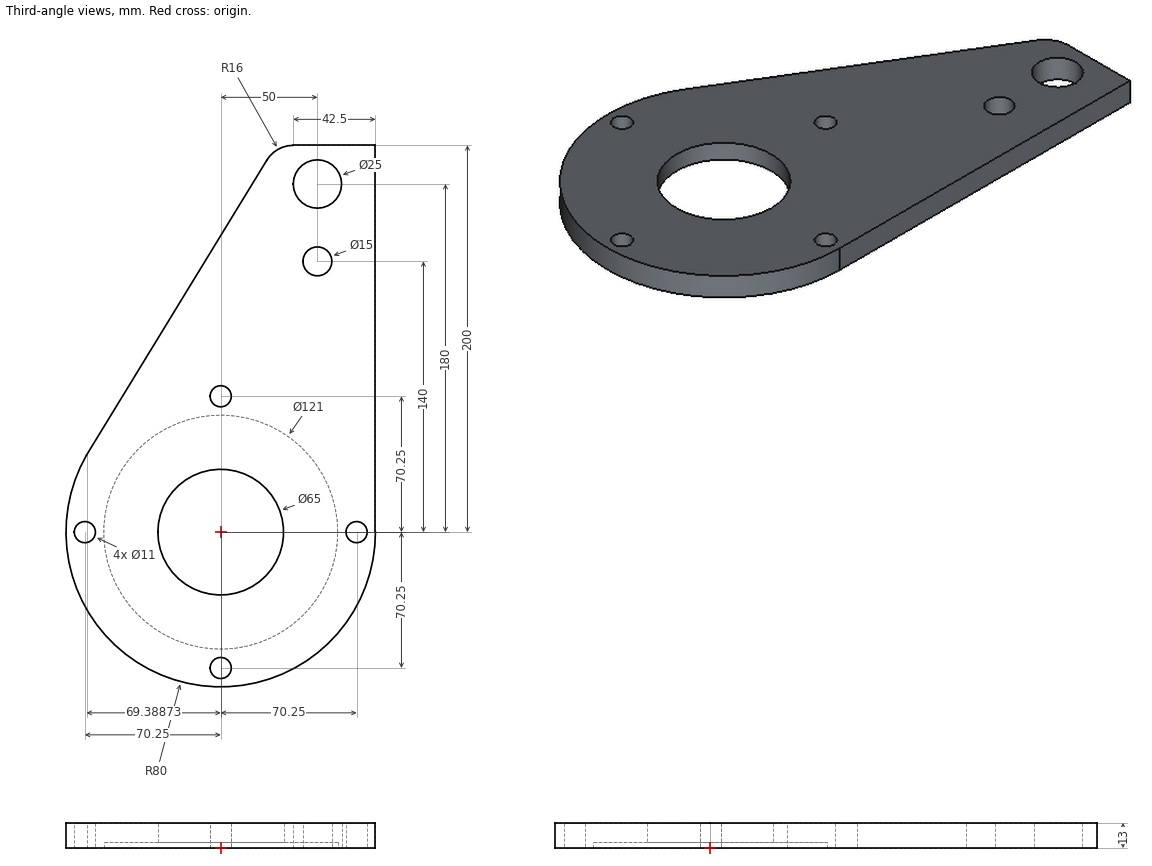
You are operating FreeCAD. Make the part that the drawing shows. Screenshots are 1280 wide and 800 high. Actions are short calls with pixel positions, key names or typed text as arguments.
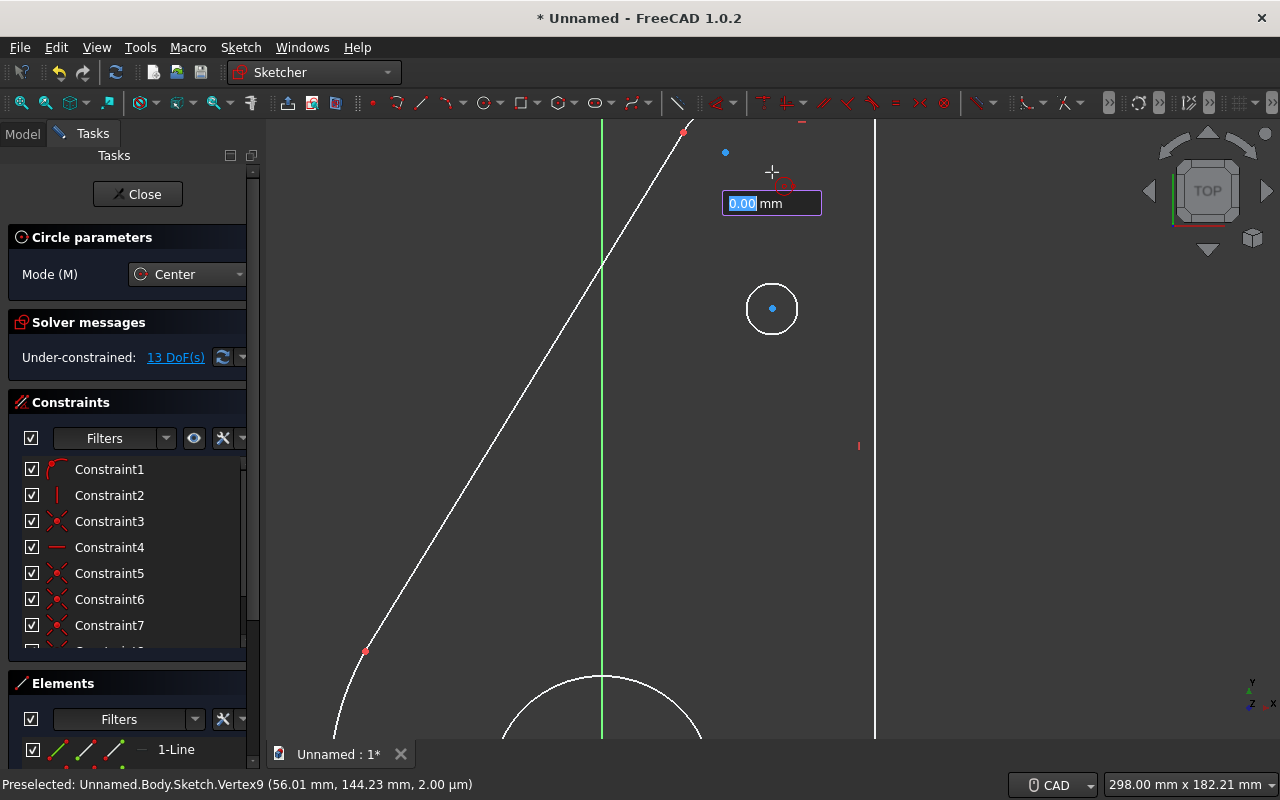
scroll(773, 309, down, 4)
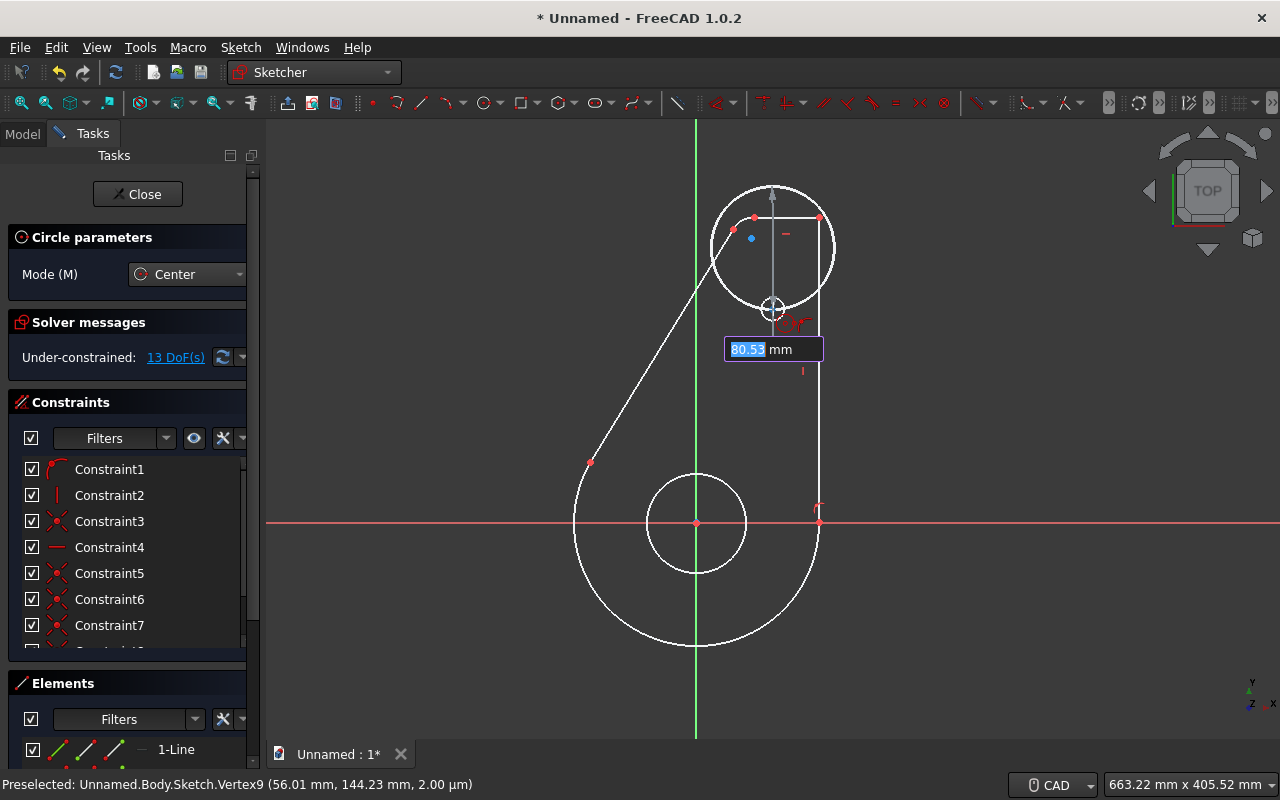
click(786, 234)
key(Escape)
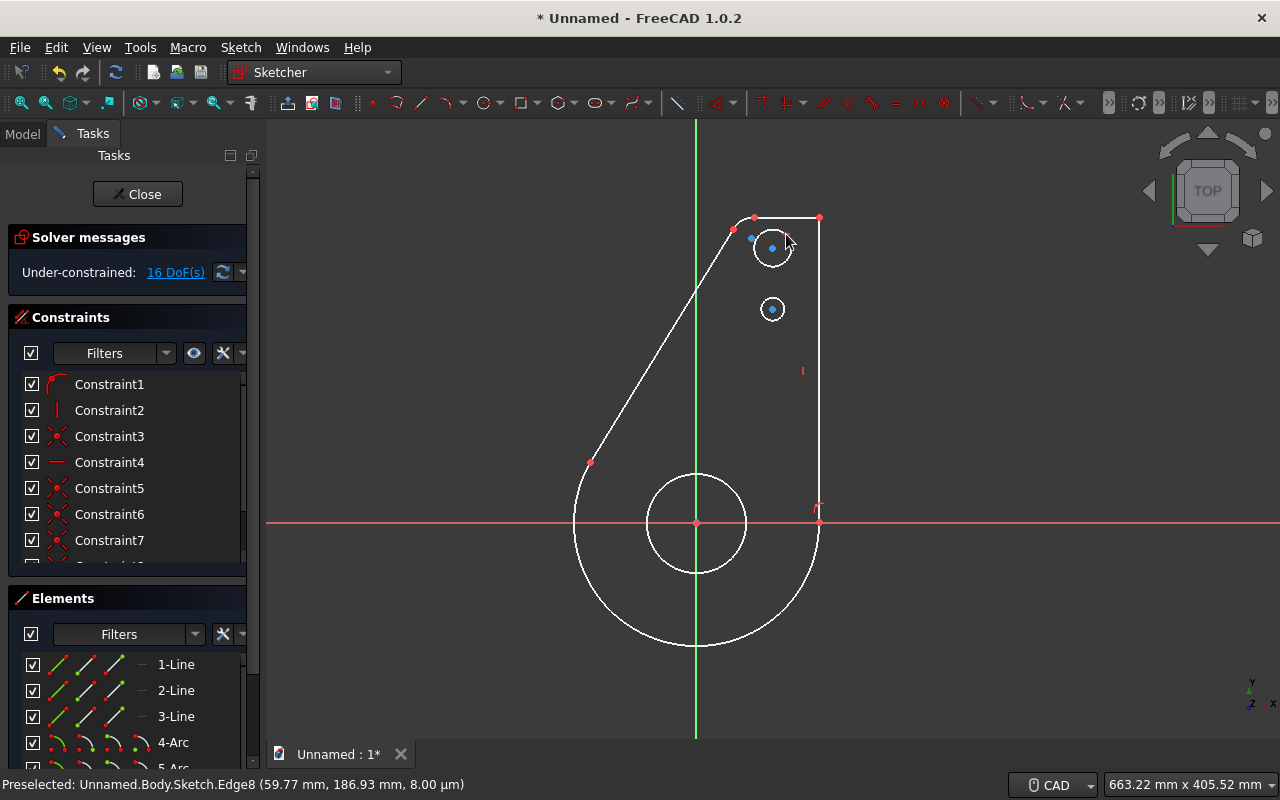
click(633, 393)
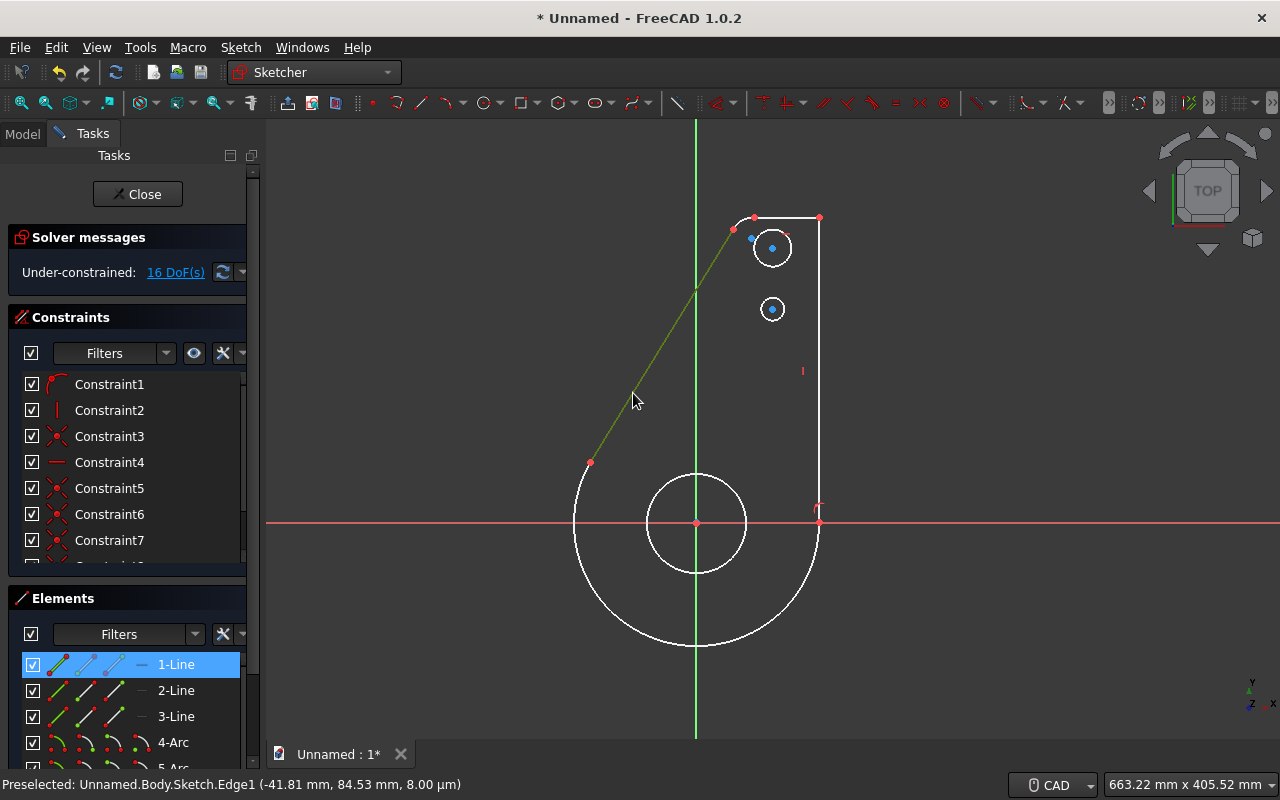
click(742, 221)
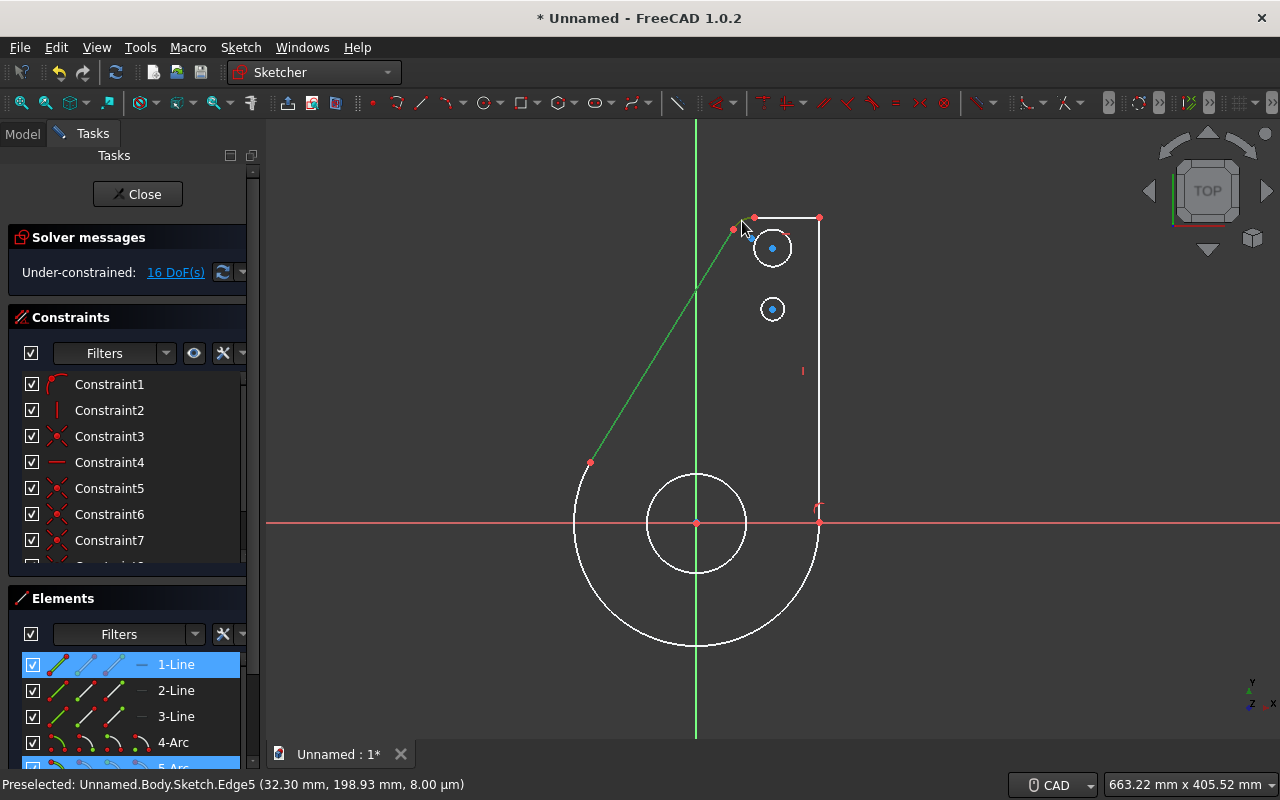
click(872, 104)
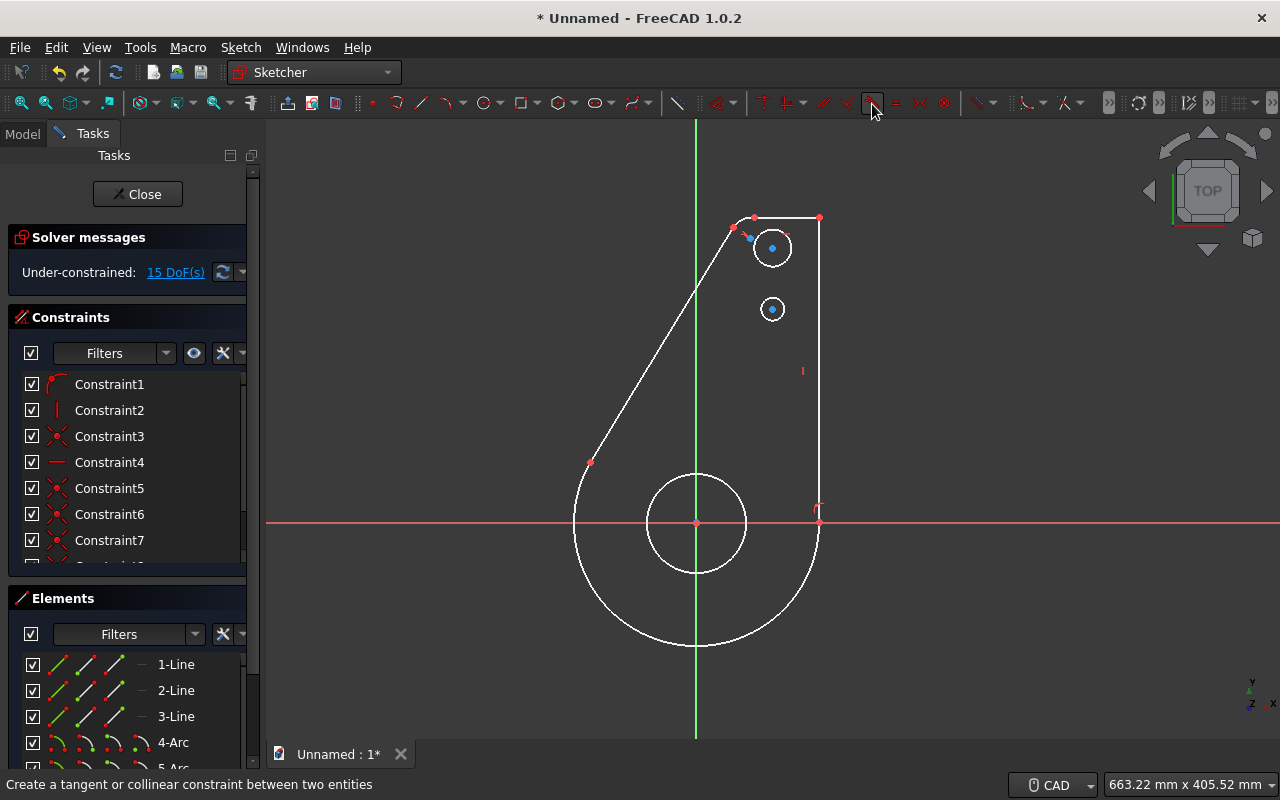
click(800, 218)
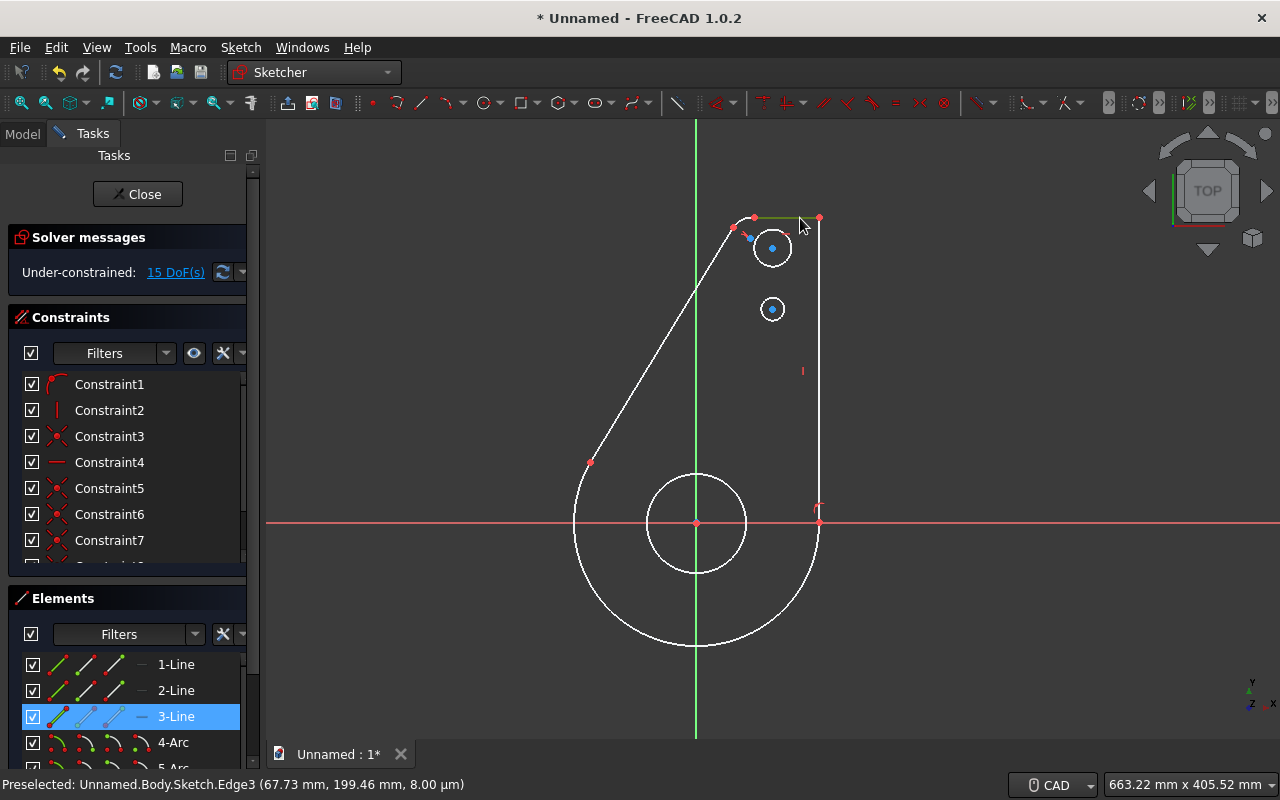
click(742, 220)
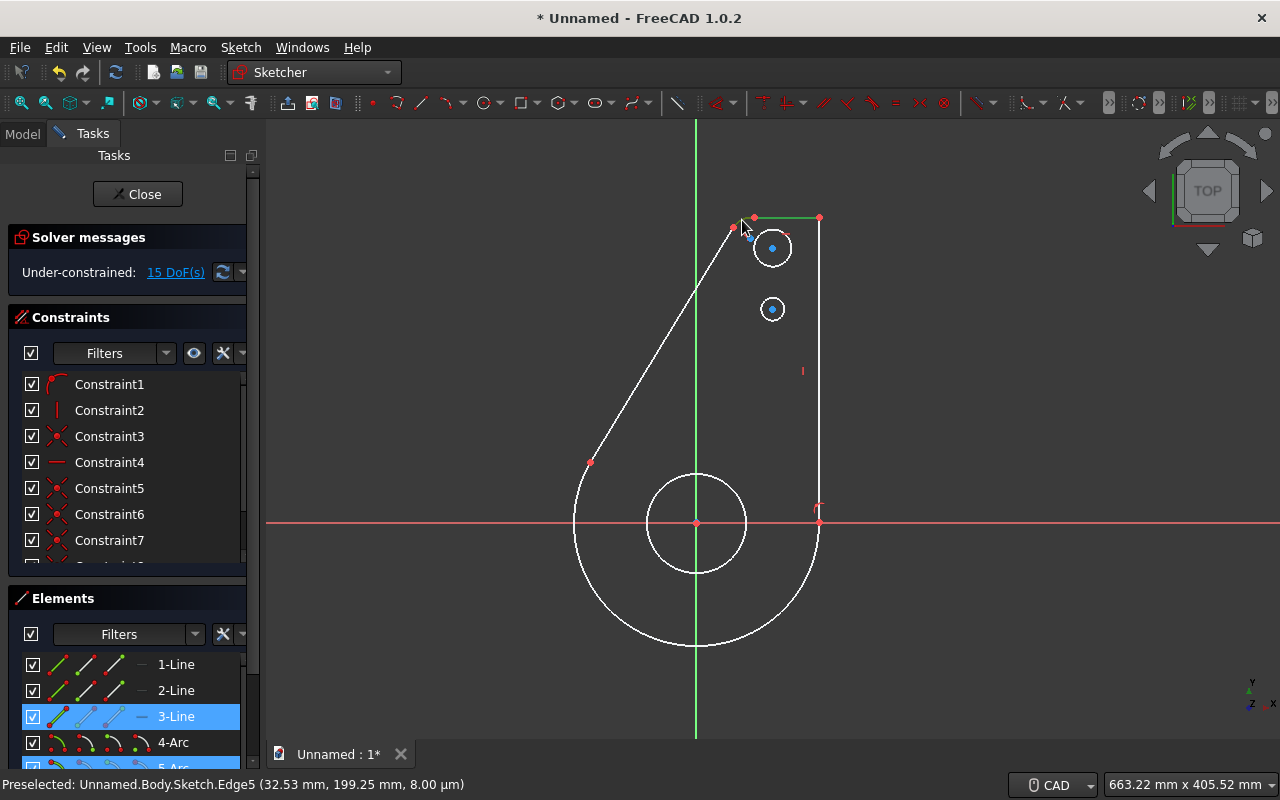
click(872, 104)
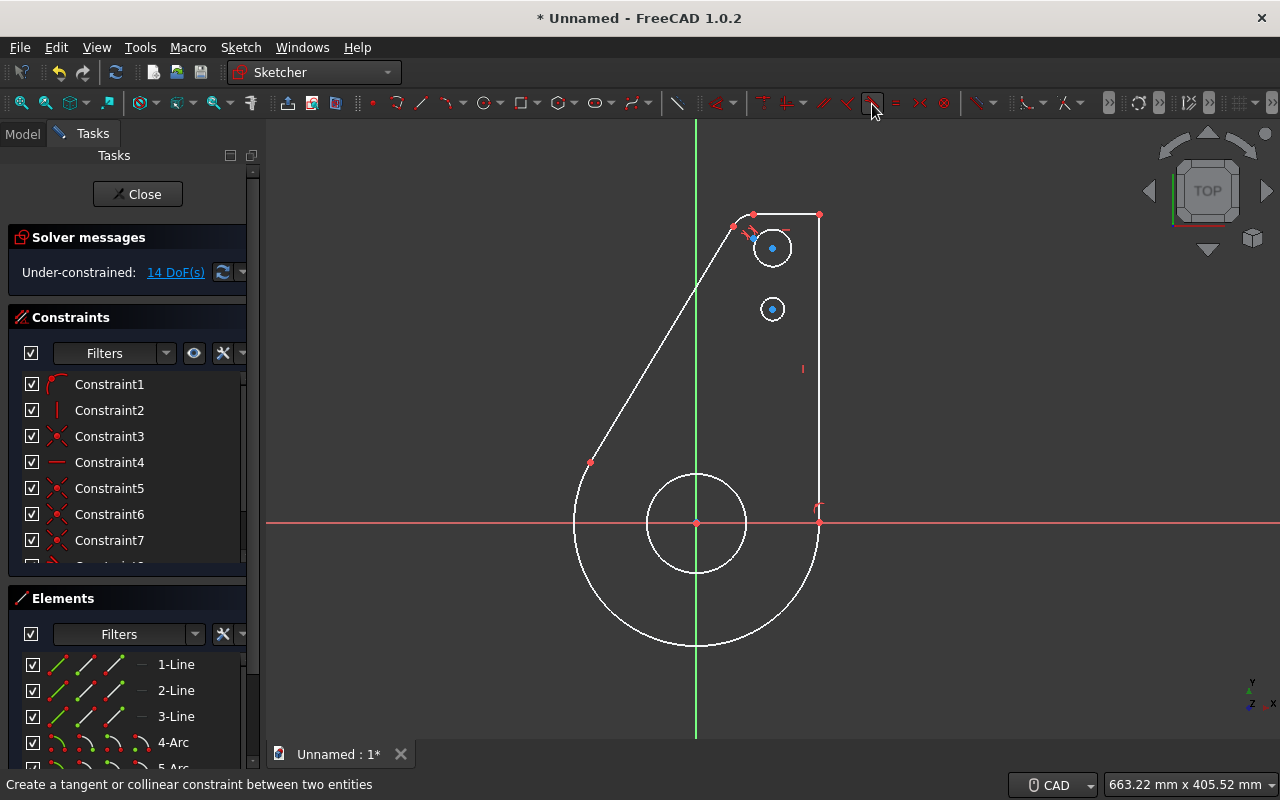
scroll(696, 523, up, 7)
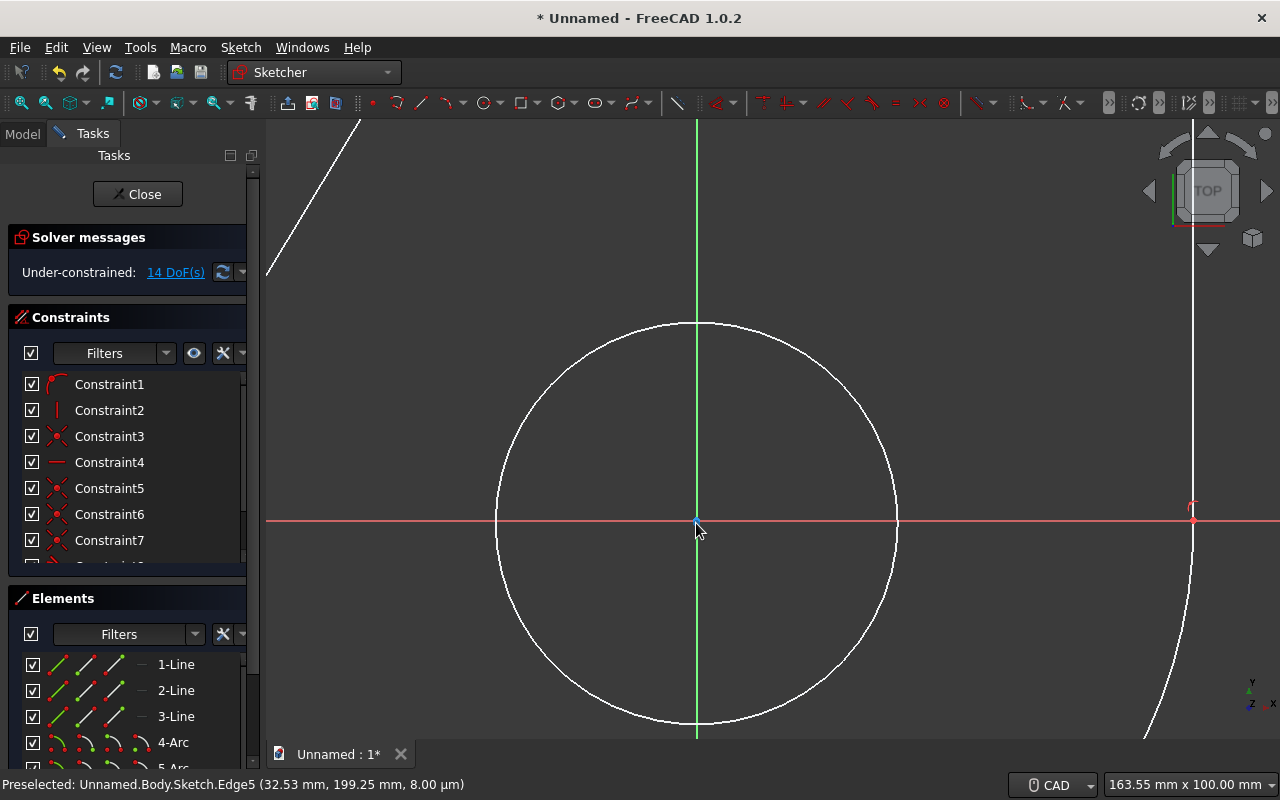
drag(687, 511, 707, 533)